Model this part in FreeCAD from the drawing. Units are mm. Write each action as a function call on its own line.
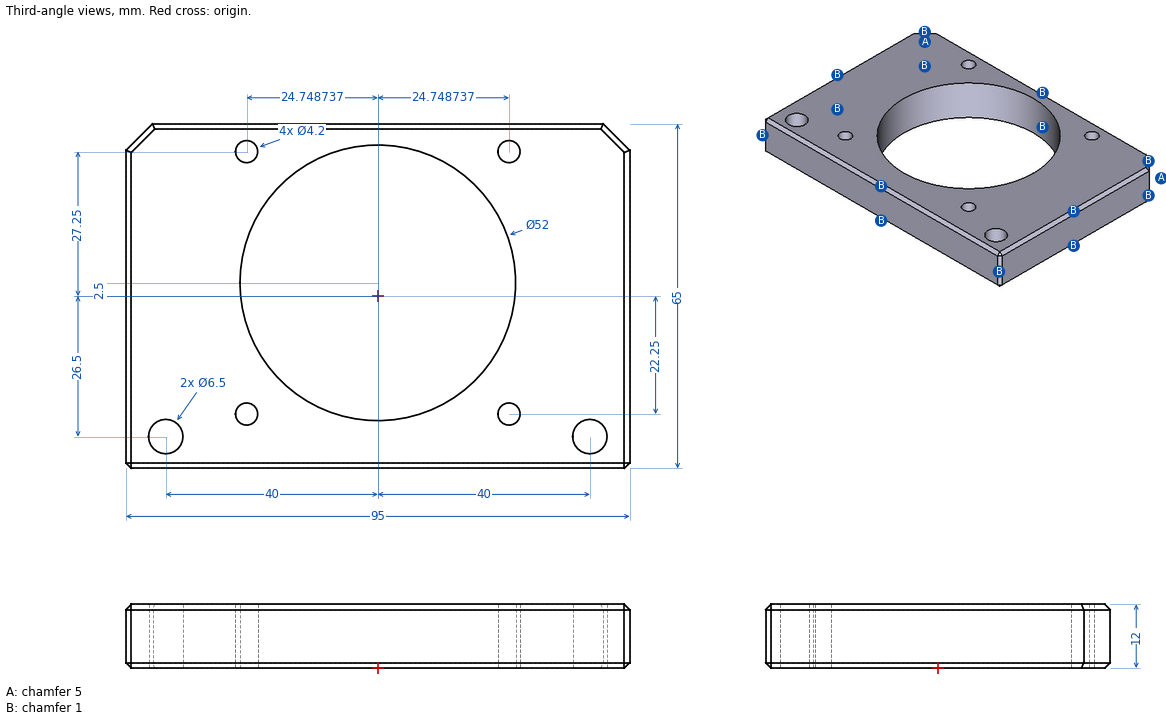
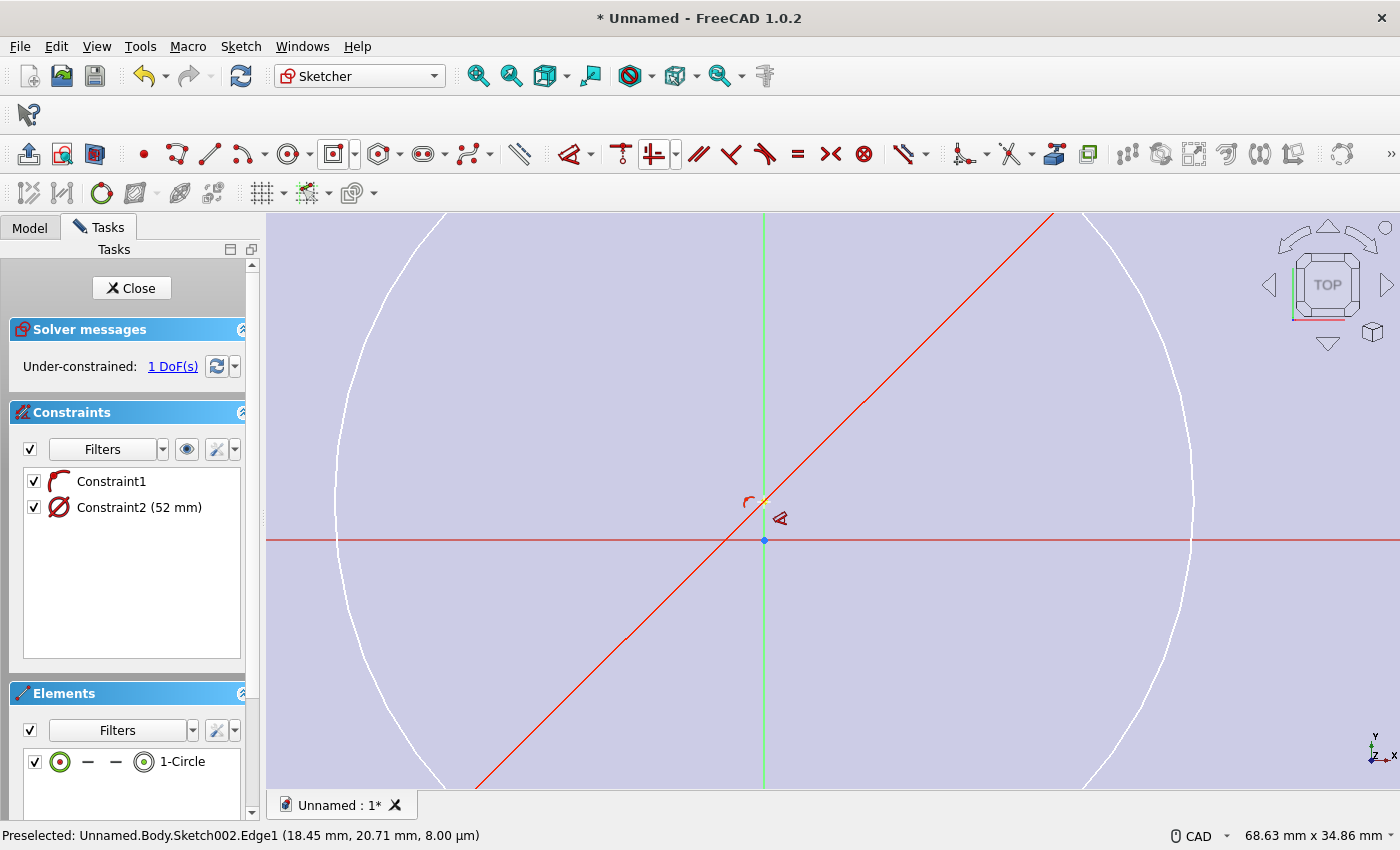
click(764, 501)
click(798, 521)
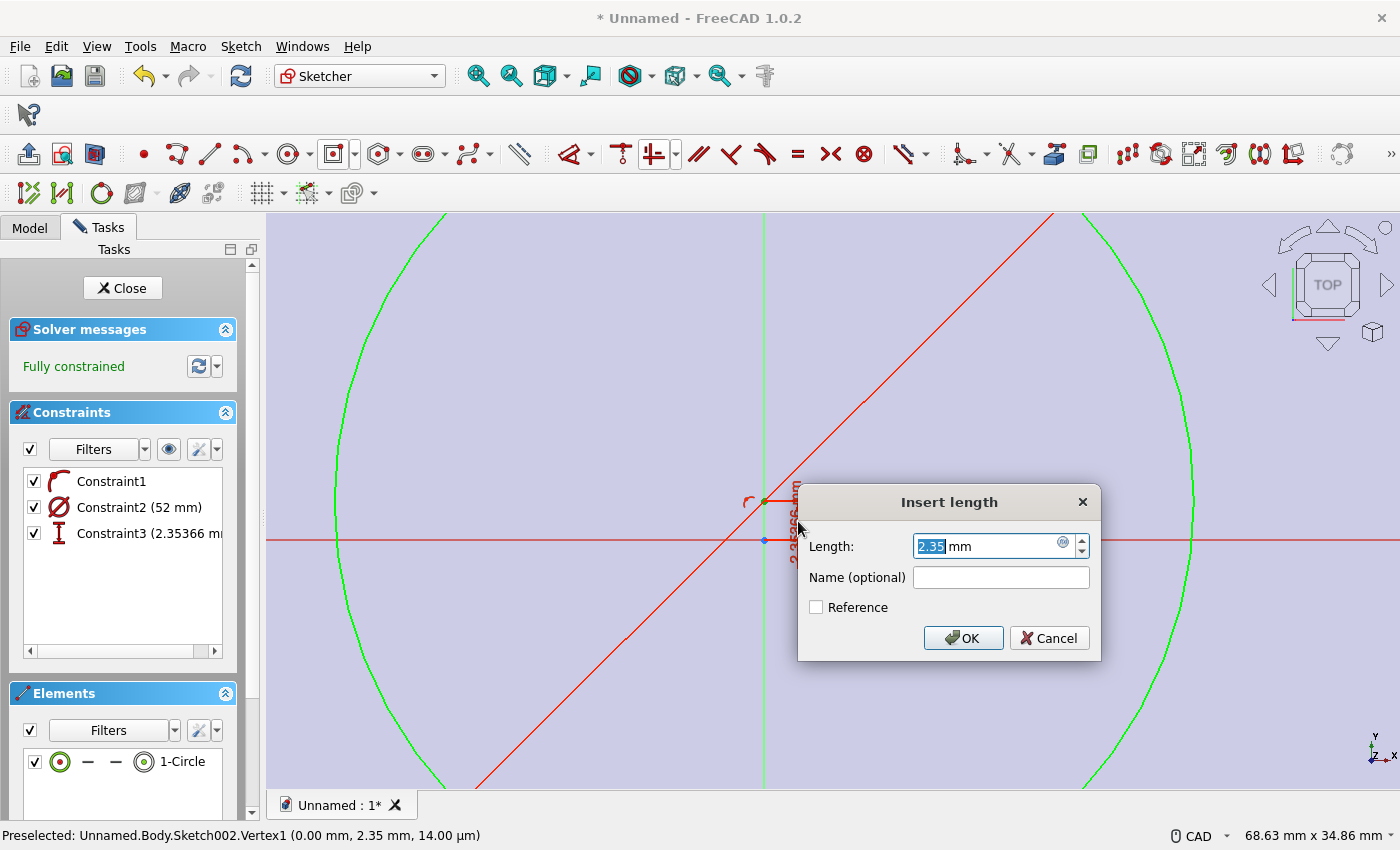
text(2.5)
key(Return)
key(Escape)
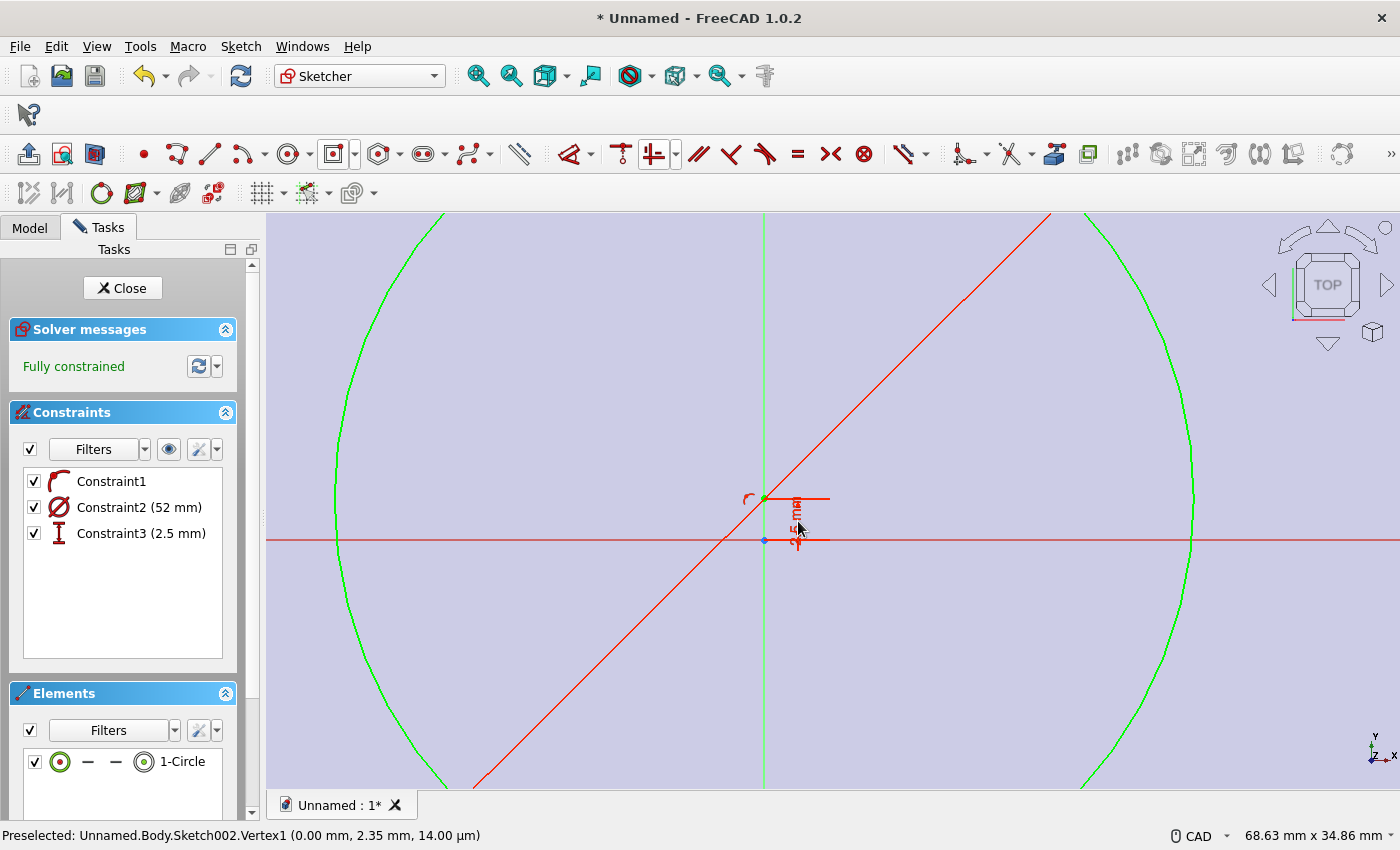
click(123, 288)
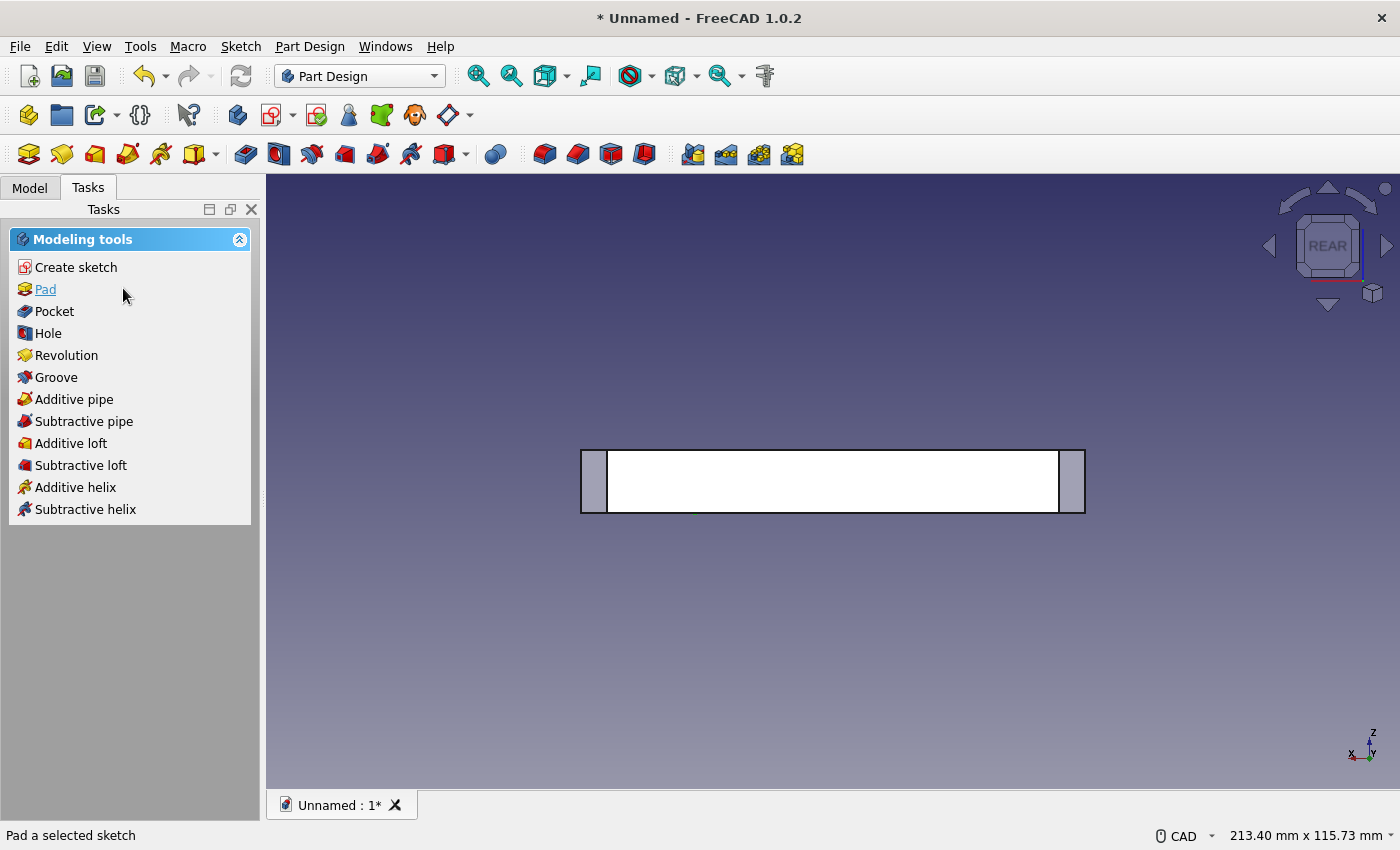
click(246, 154)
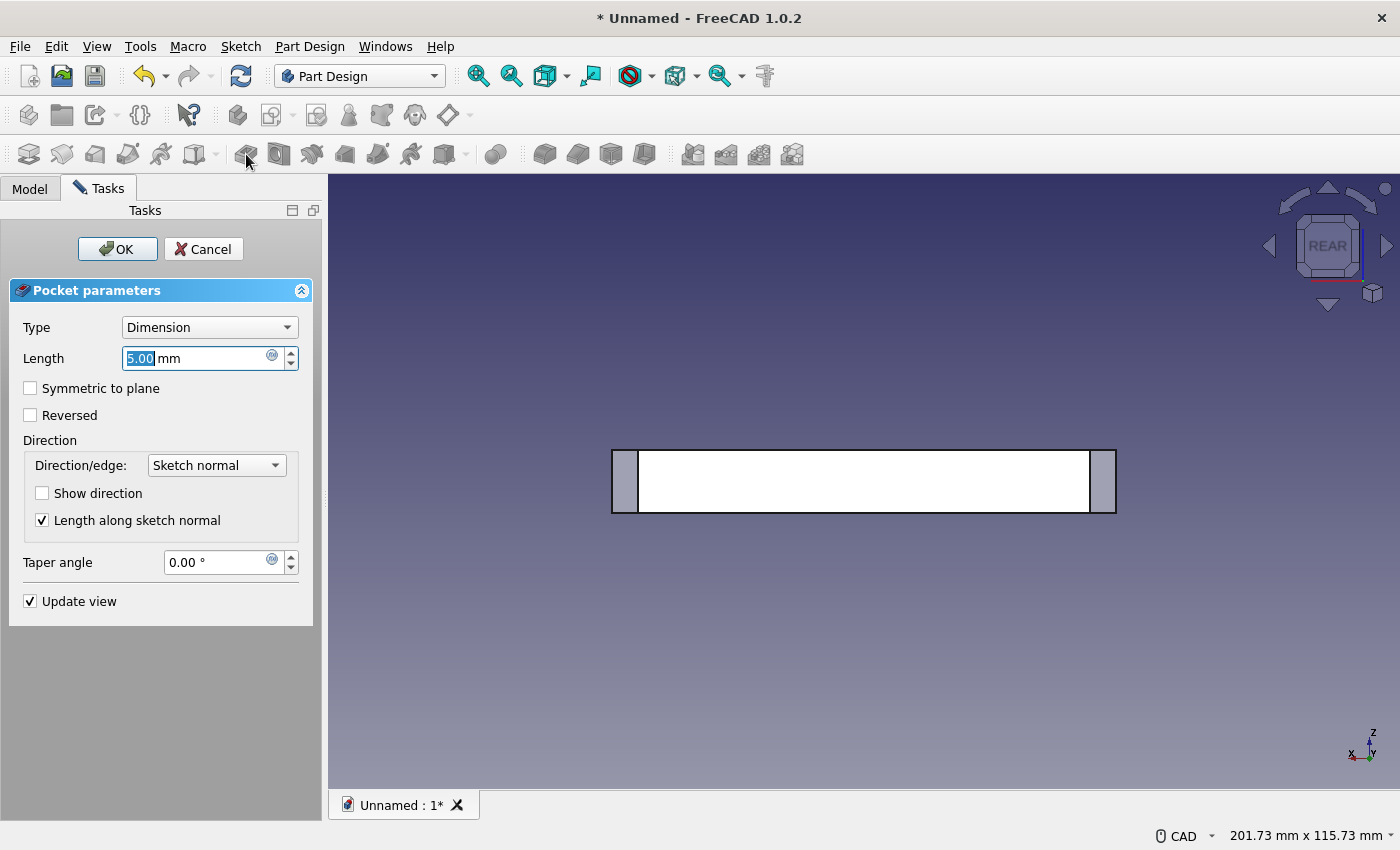
click(210, 328)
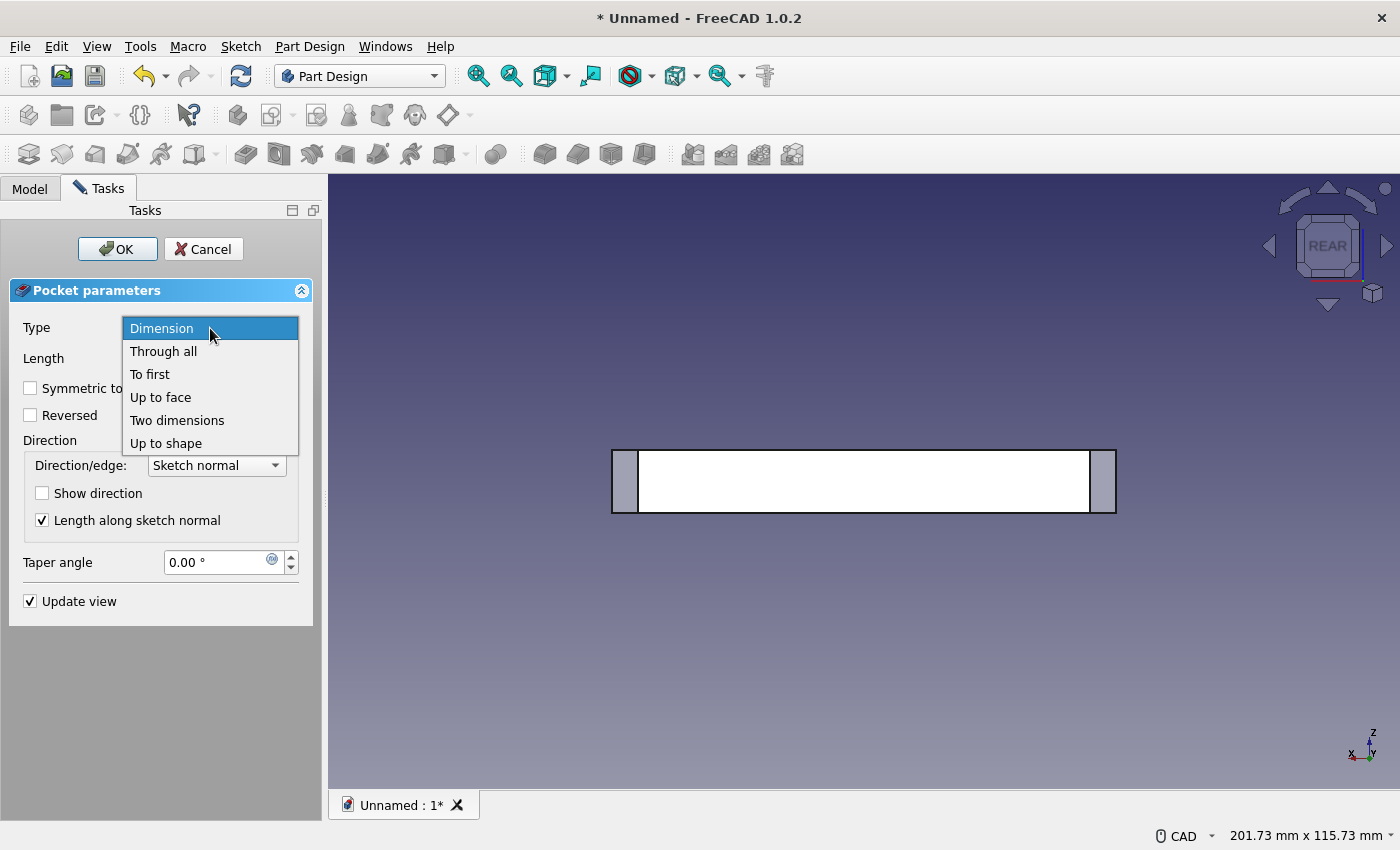
click(208, 352)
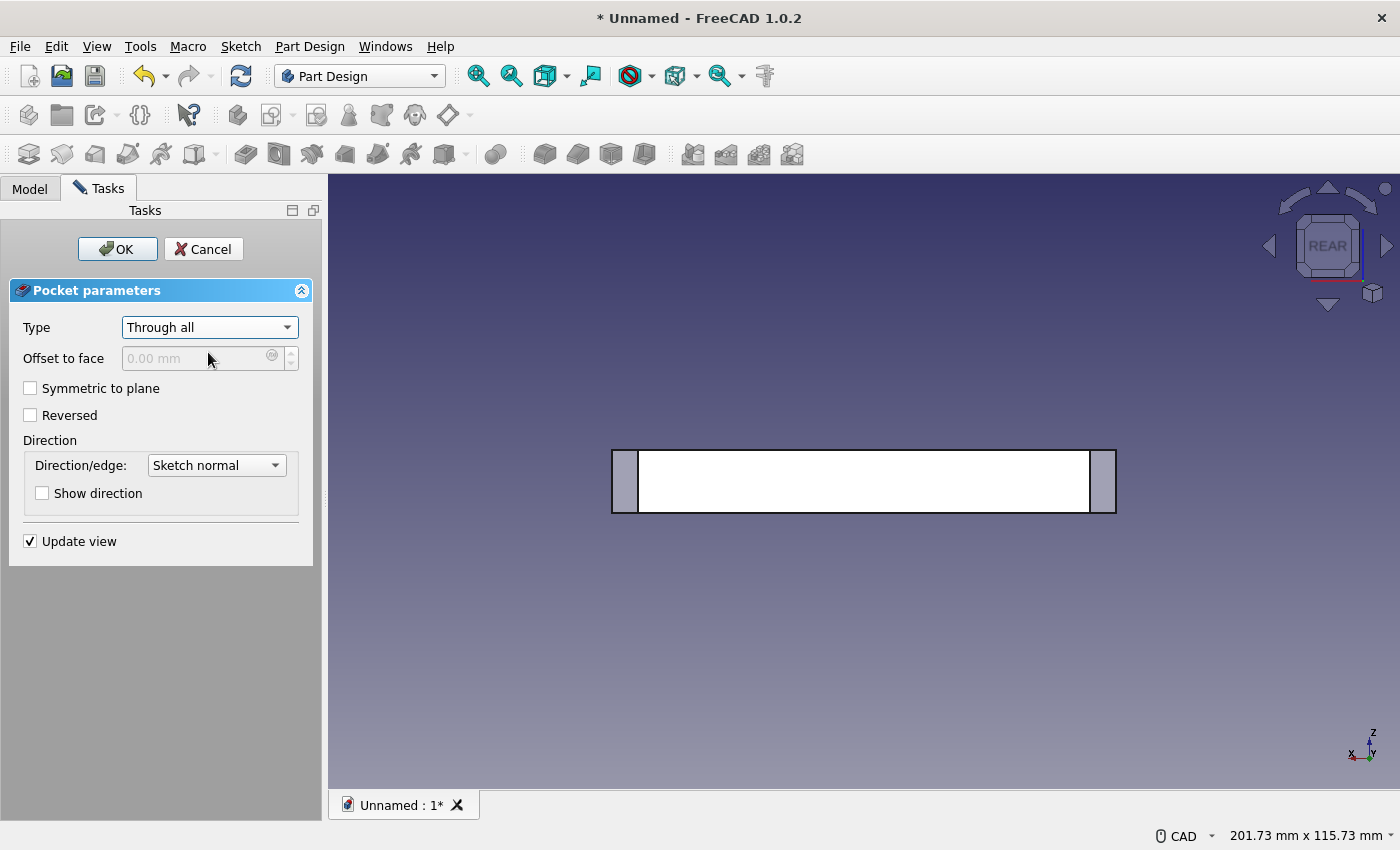
click(31, 415)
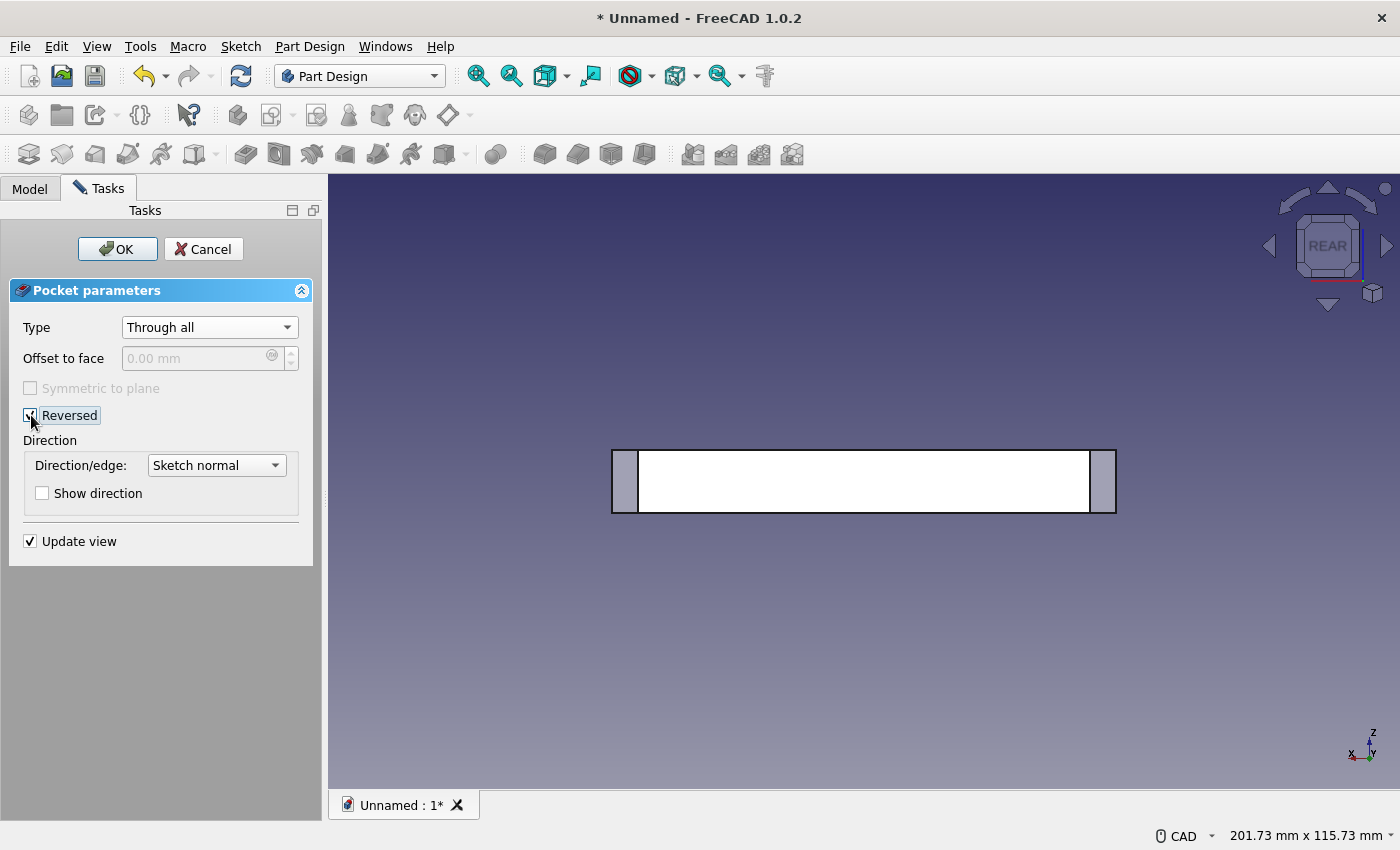
click(118, 249)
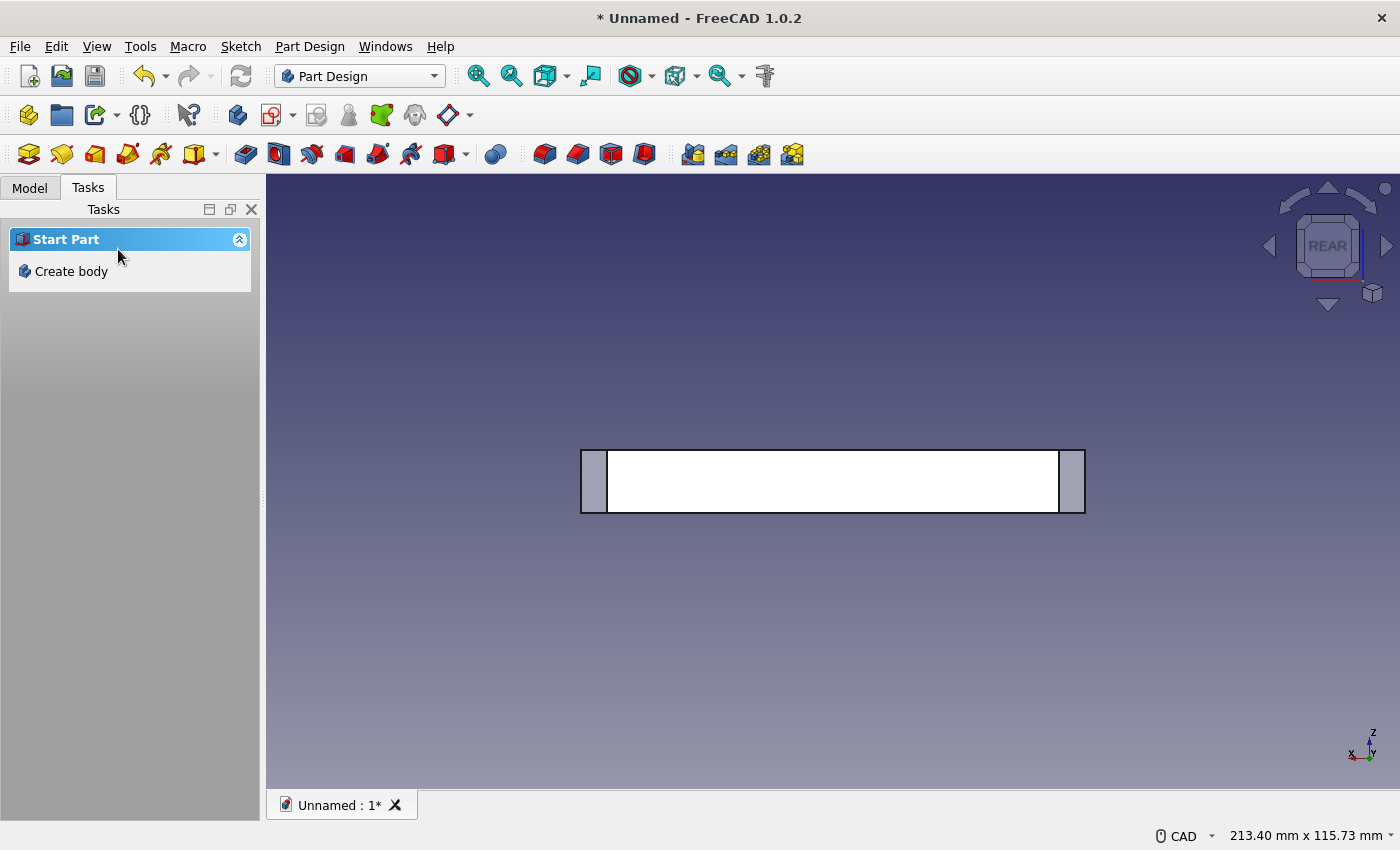
key(v)
key(f)